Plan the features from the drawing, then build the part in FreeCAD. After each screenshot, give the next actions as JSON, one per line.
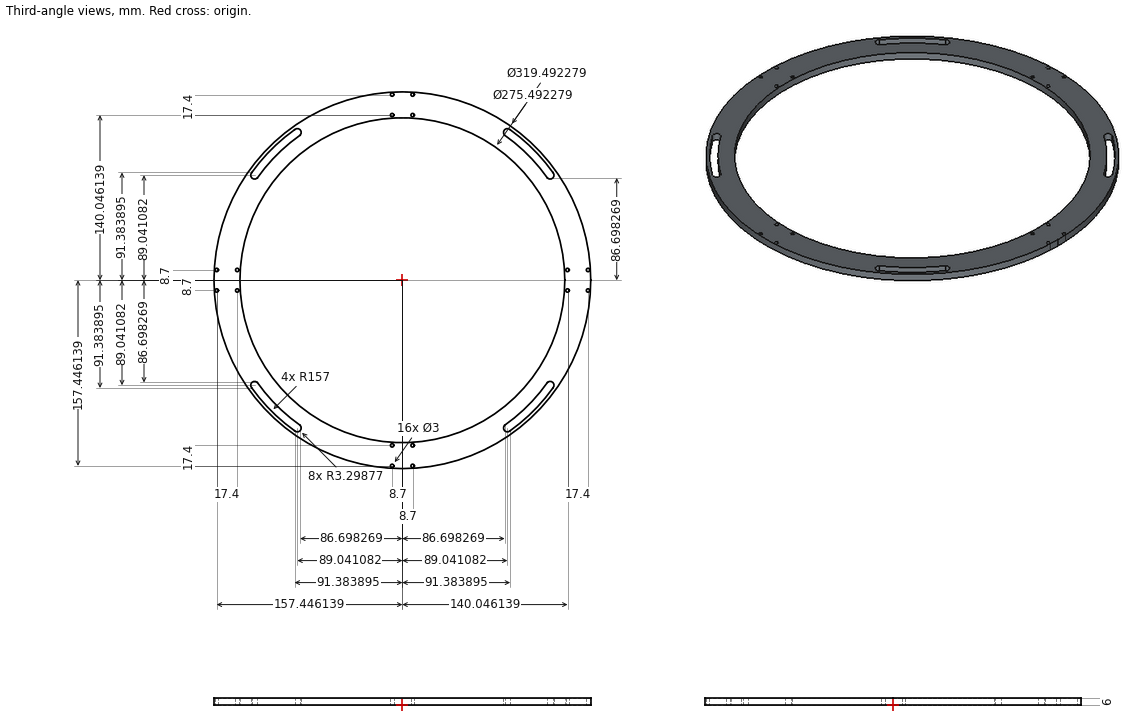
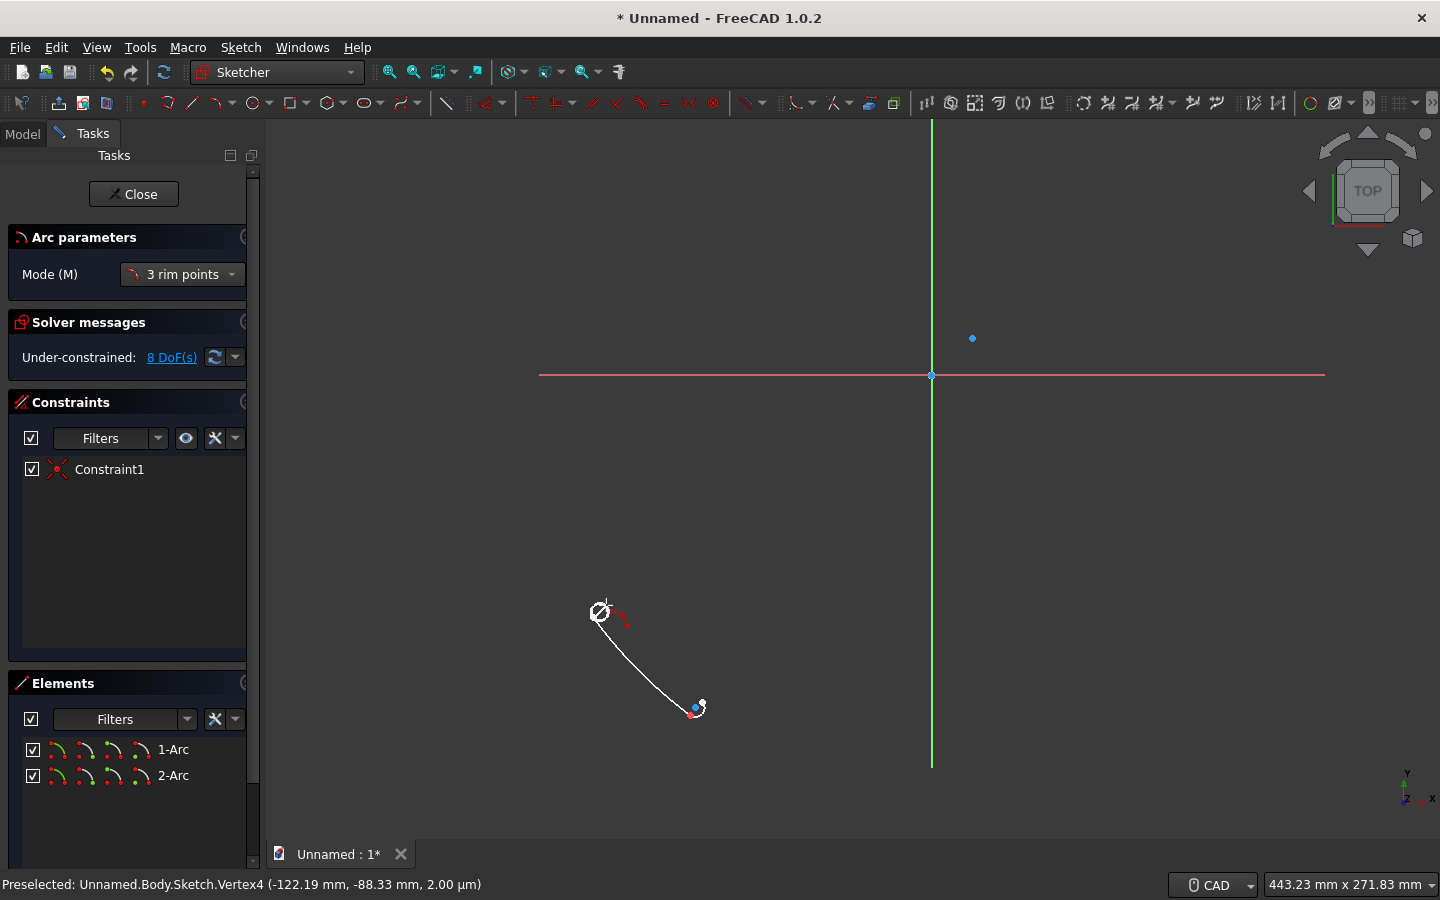
{"action": "scroll", "coordinate": [594, 605], "scroll_direction": "up", "scroll_amount": 3}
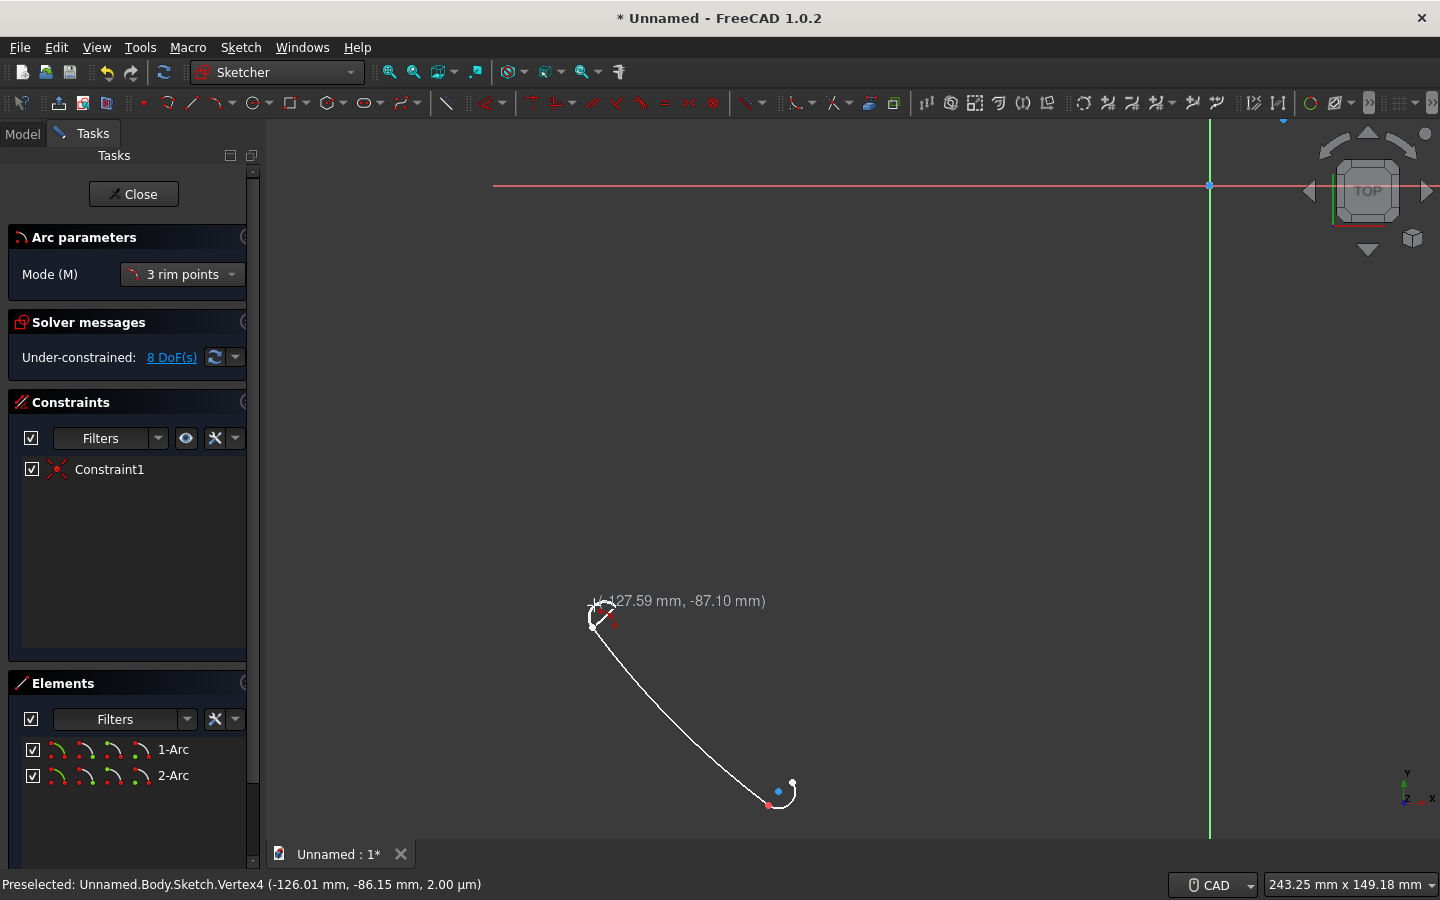
{"action": "left_click", "coordinate": [593, 604]}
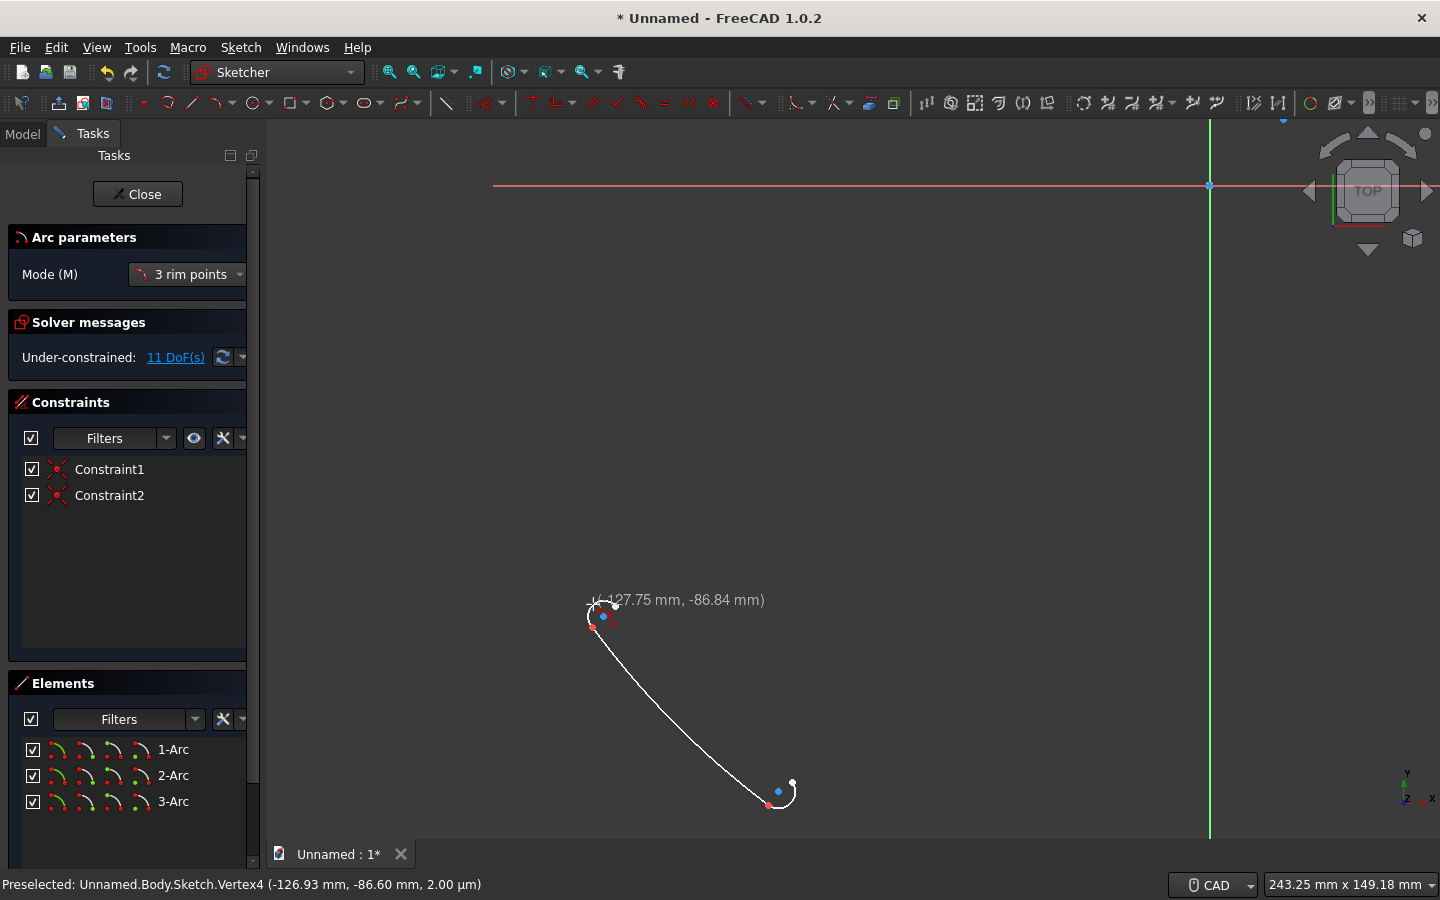
{"action": "left_click", "coordinate": [616, 606]}
{"action": "left_click", "coordinate": [792, 782]}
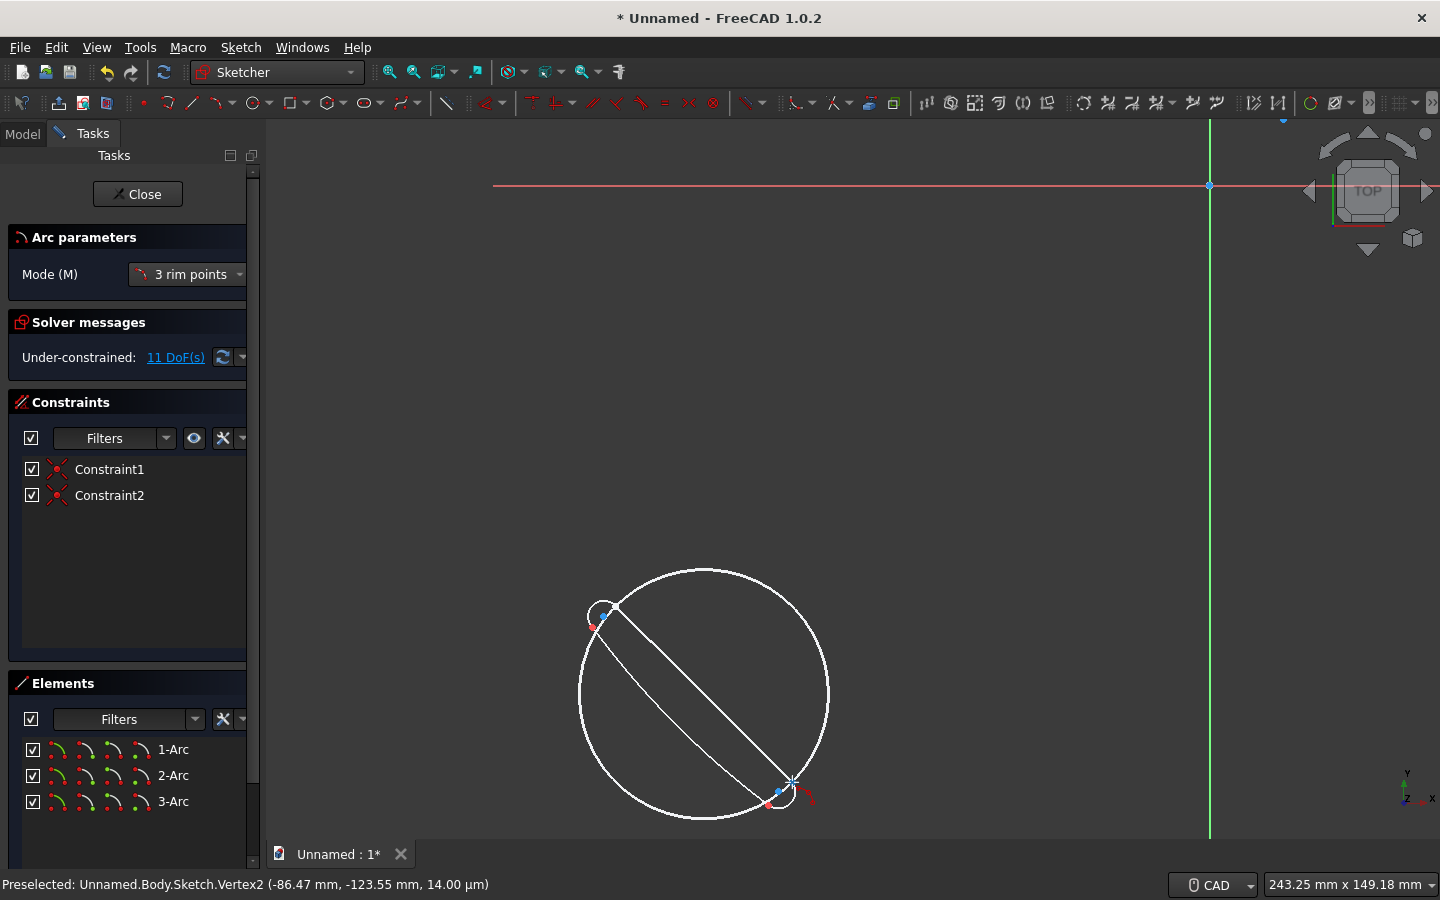
{"action": "scroll", "coordinate": [696, 700], "scroll_direction": "up", "scroll_amount": 2}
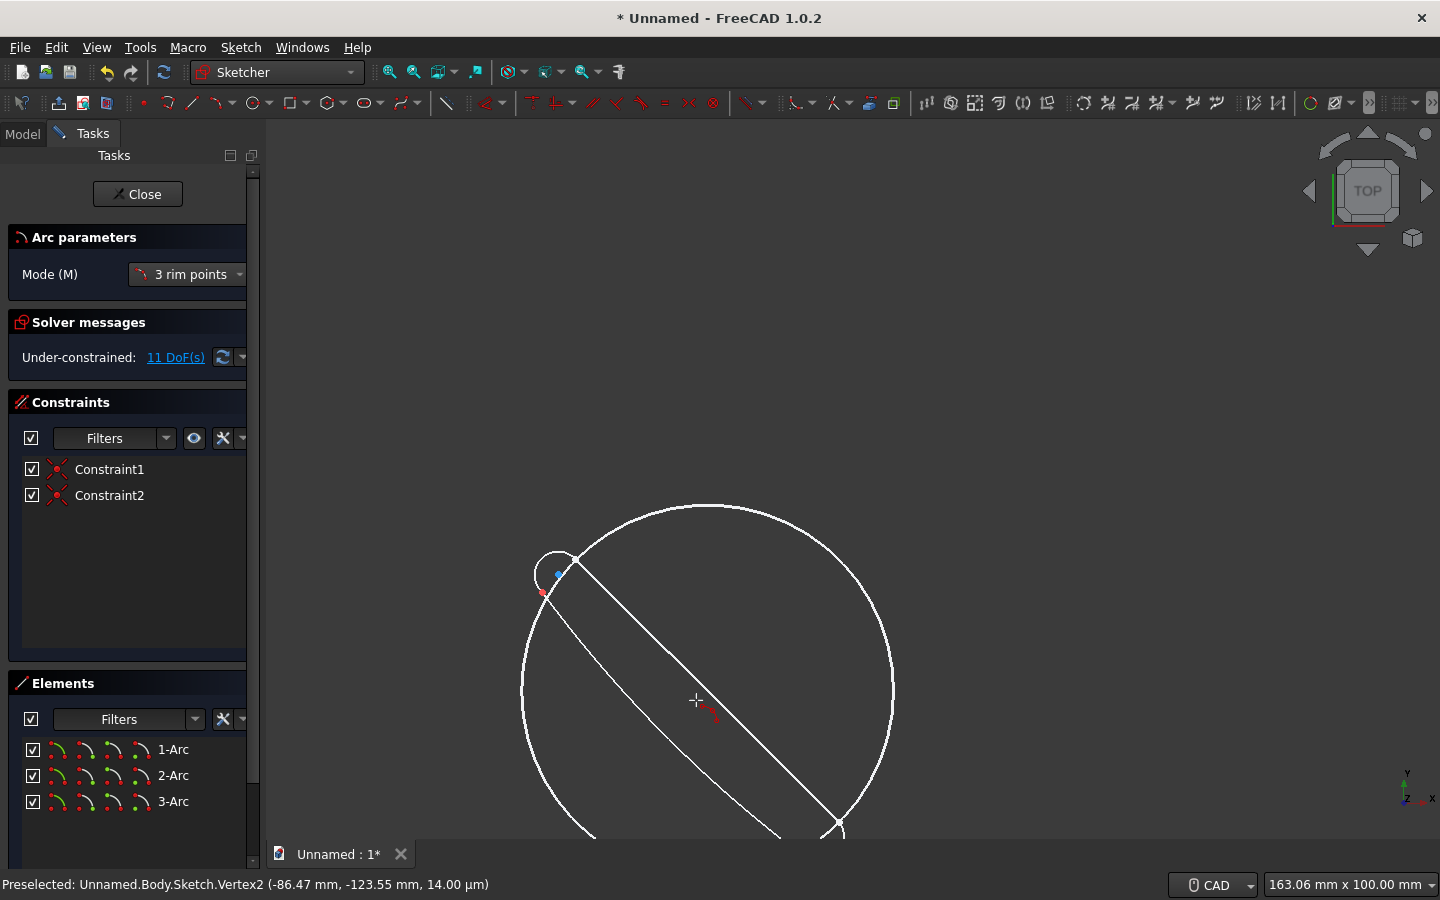
{"action": "left_click", "coordinate": [696, 699]}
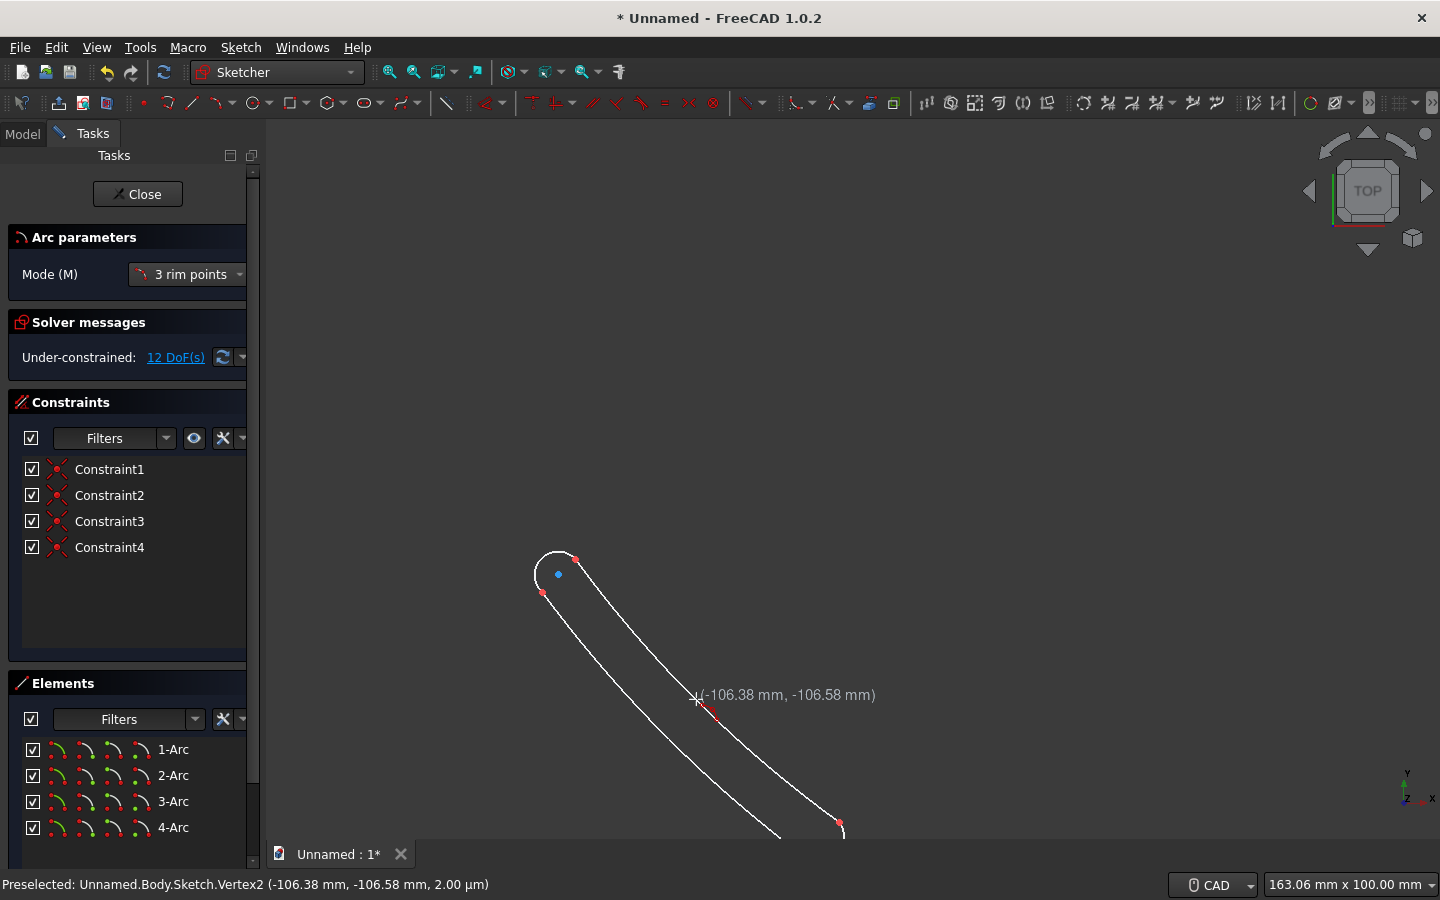
{"action": "scroll", "coordinate": [613, 617], "scroll_direction": "down", "scroll_amount": 8}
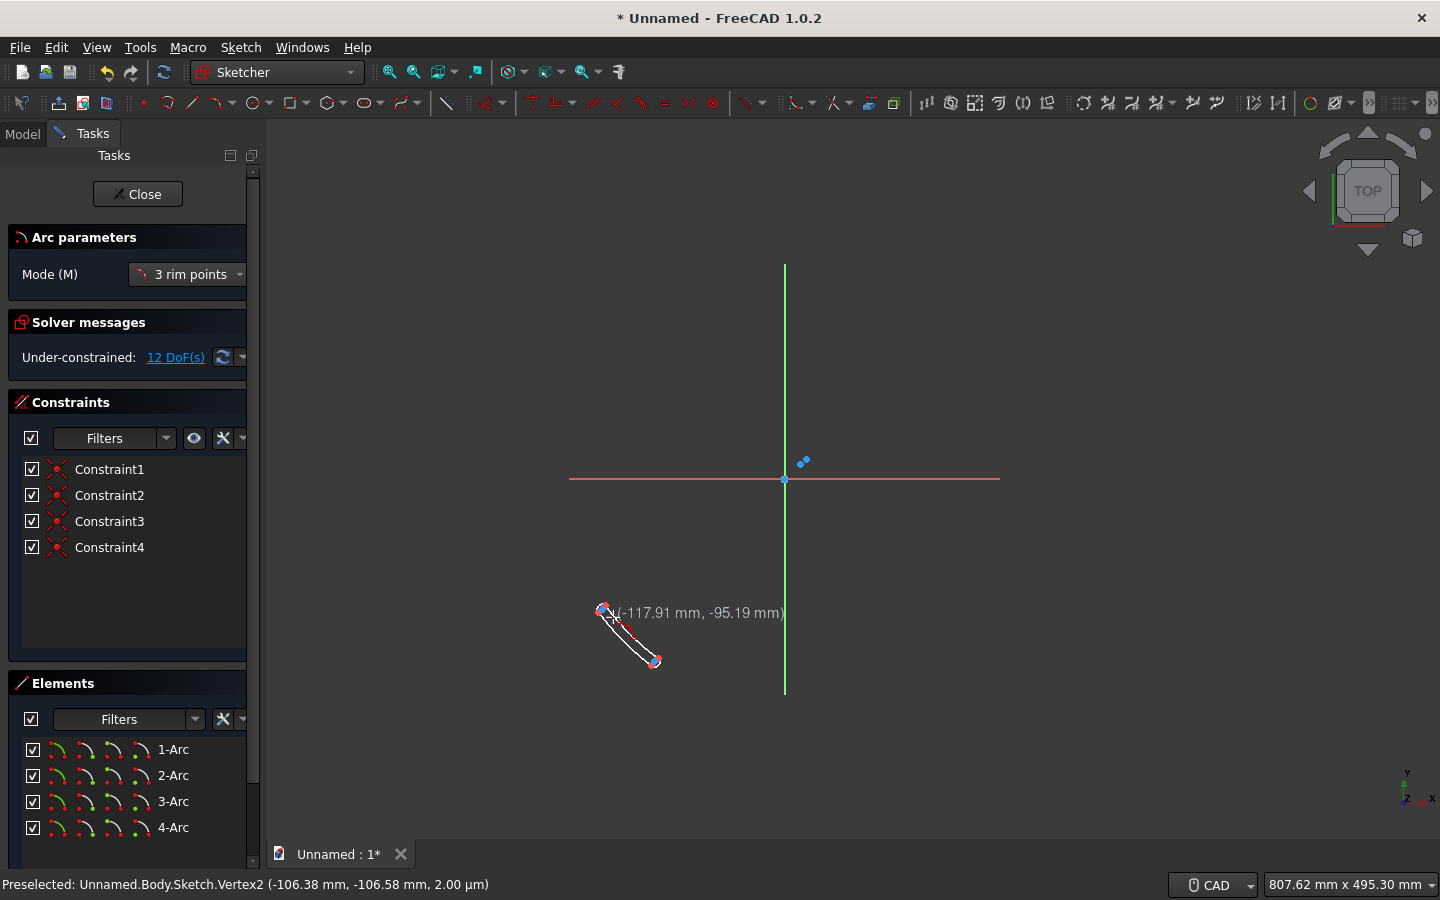
{"action": "left_click", "coordinate": [963, 605]}
{"action": "left_click", "coordinate": [970, 612]}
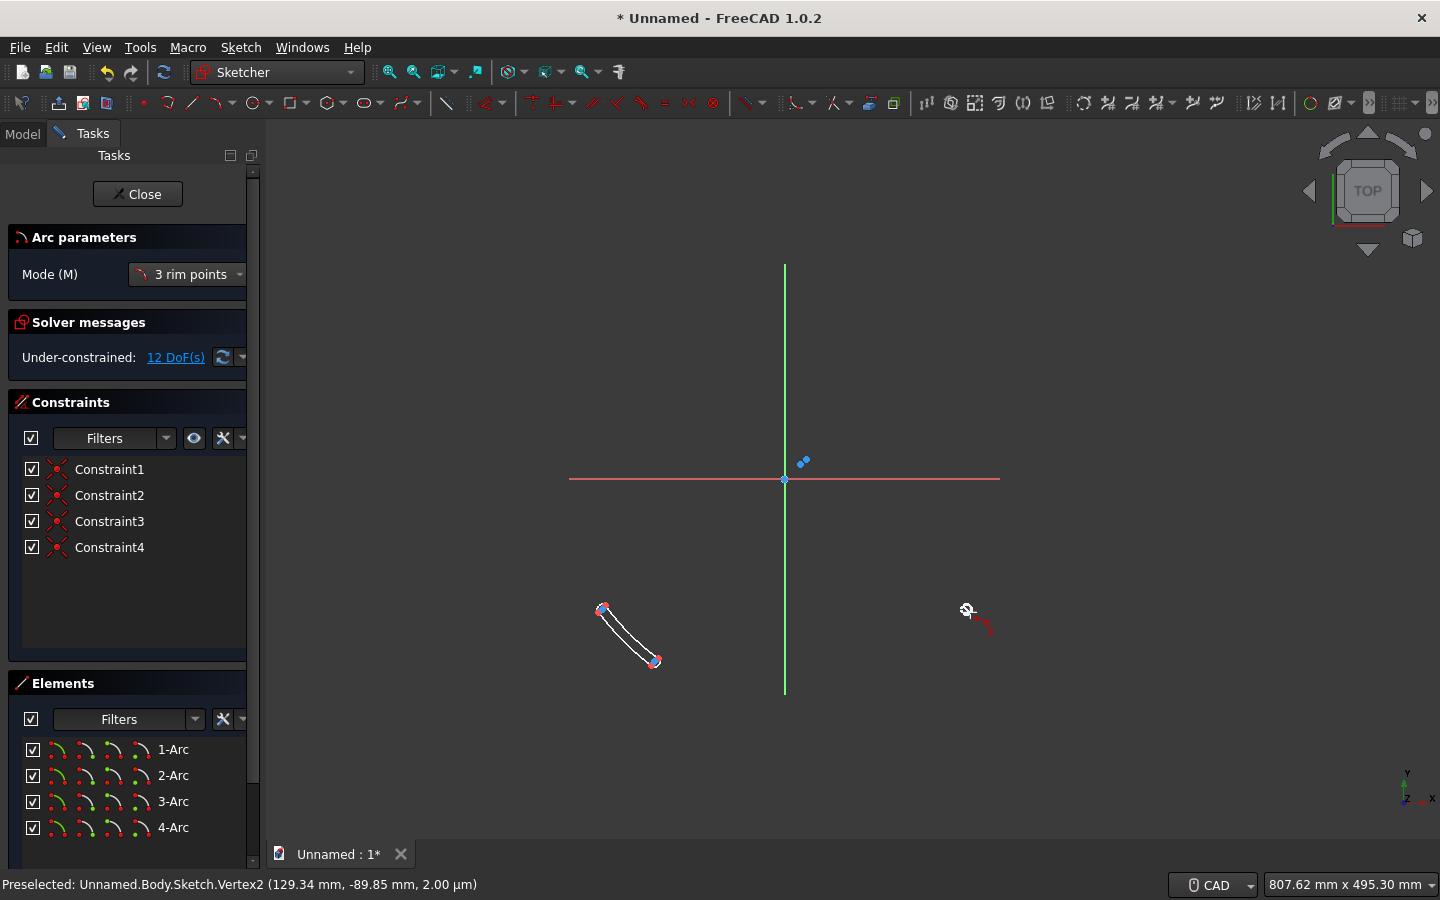
{"action": "scroll", "coordinate": [970, 605], "scroll_direction": "up", "scroll_amount": 6}